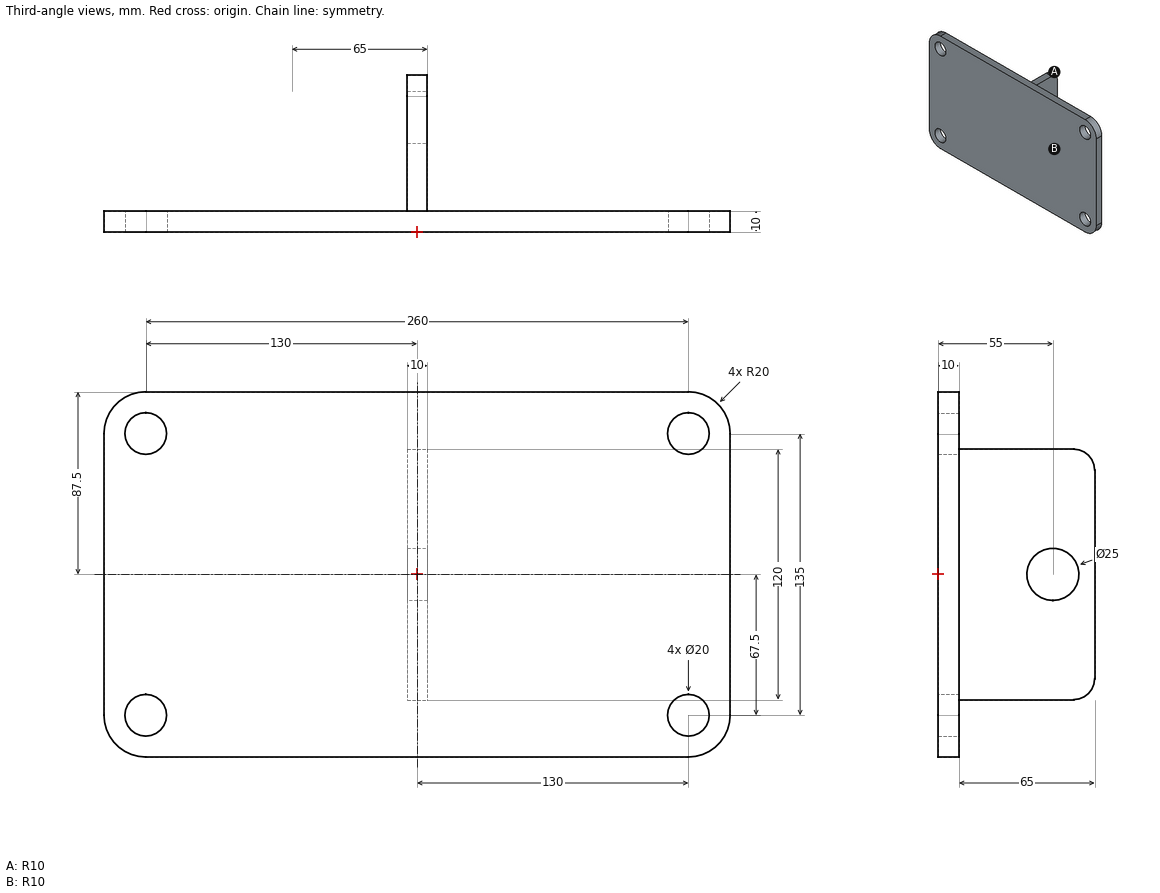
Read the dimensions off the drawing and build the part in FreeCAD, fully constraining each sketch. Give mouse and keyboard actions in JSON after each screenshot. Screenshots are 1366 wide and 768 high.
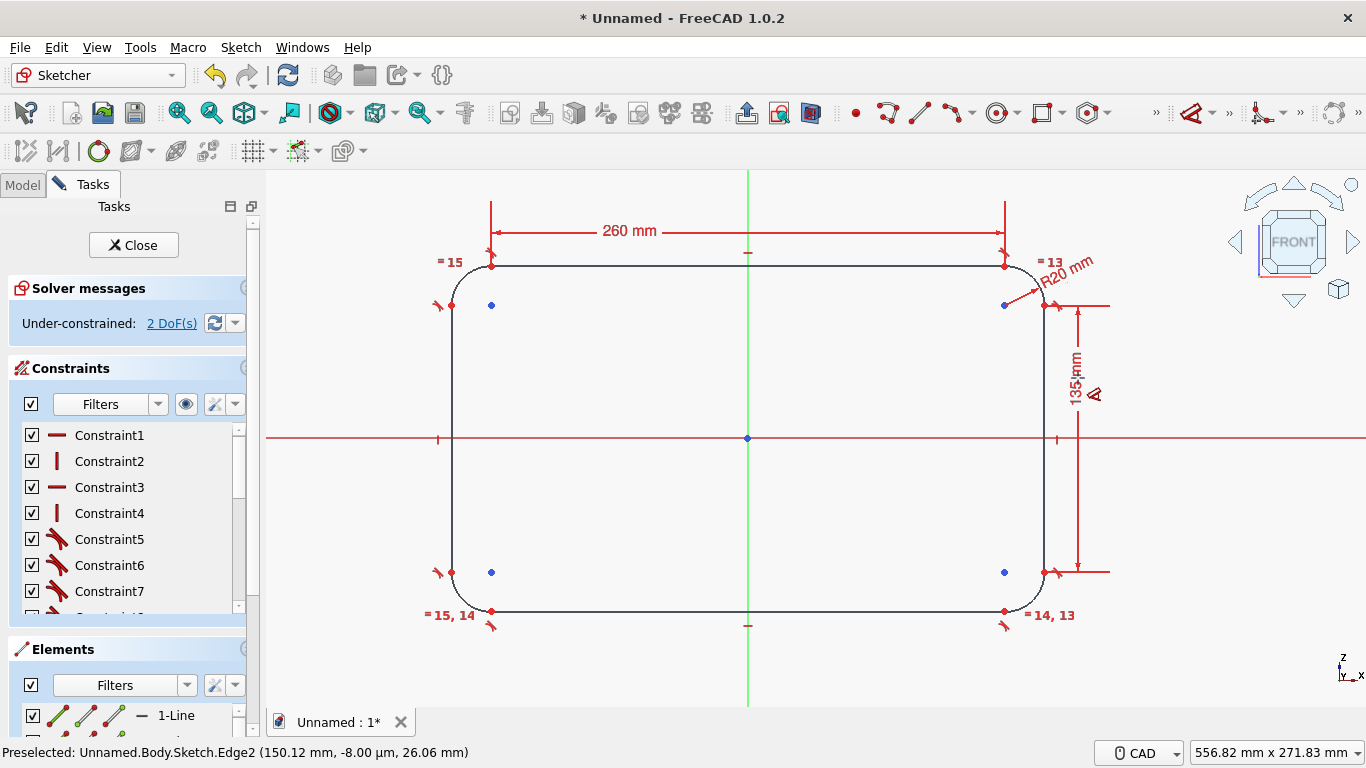
{"action": "left_click", "coordinate": [491, 266]}
{"action": "left_click", "coordinate": [530, 232]}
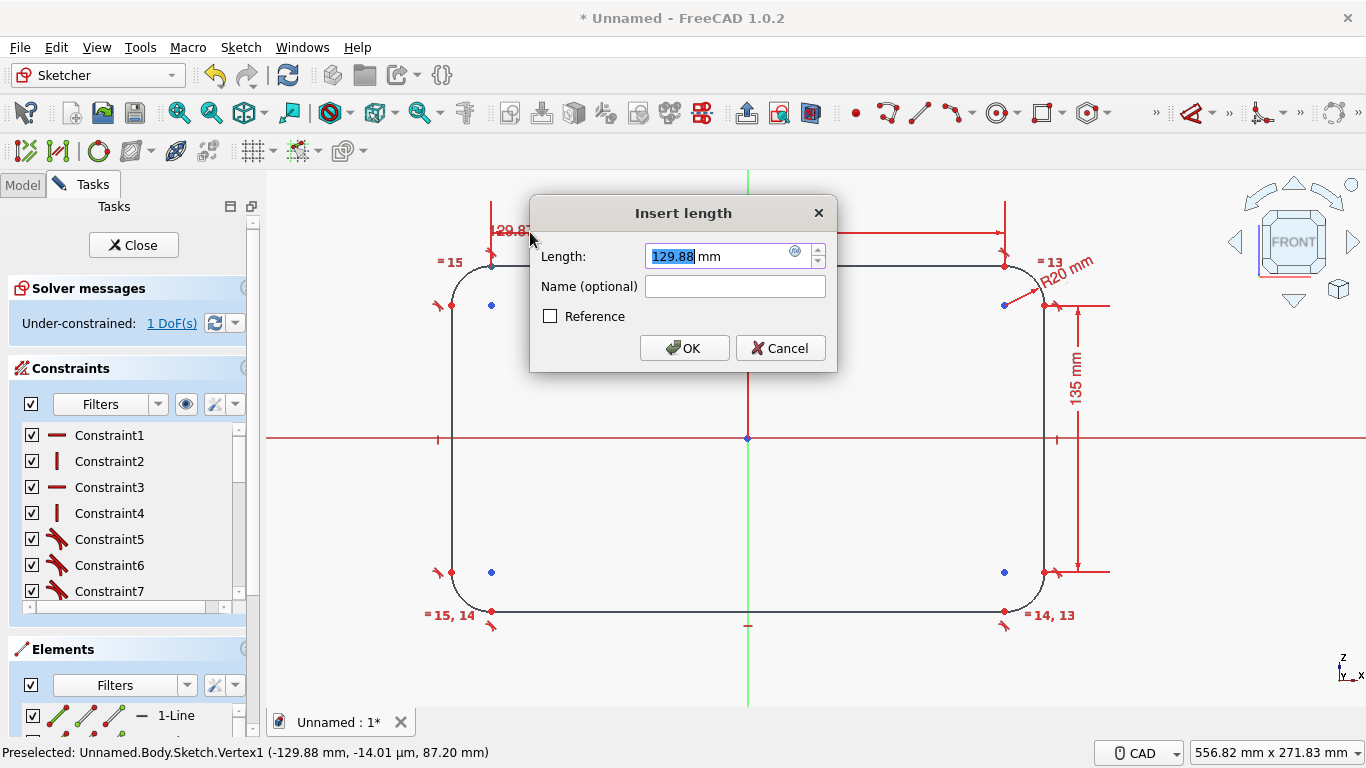
{"action": "type", "text": "130"}
{"action": "key", "text": "Return"}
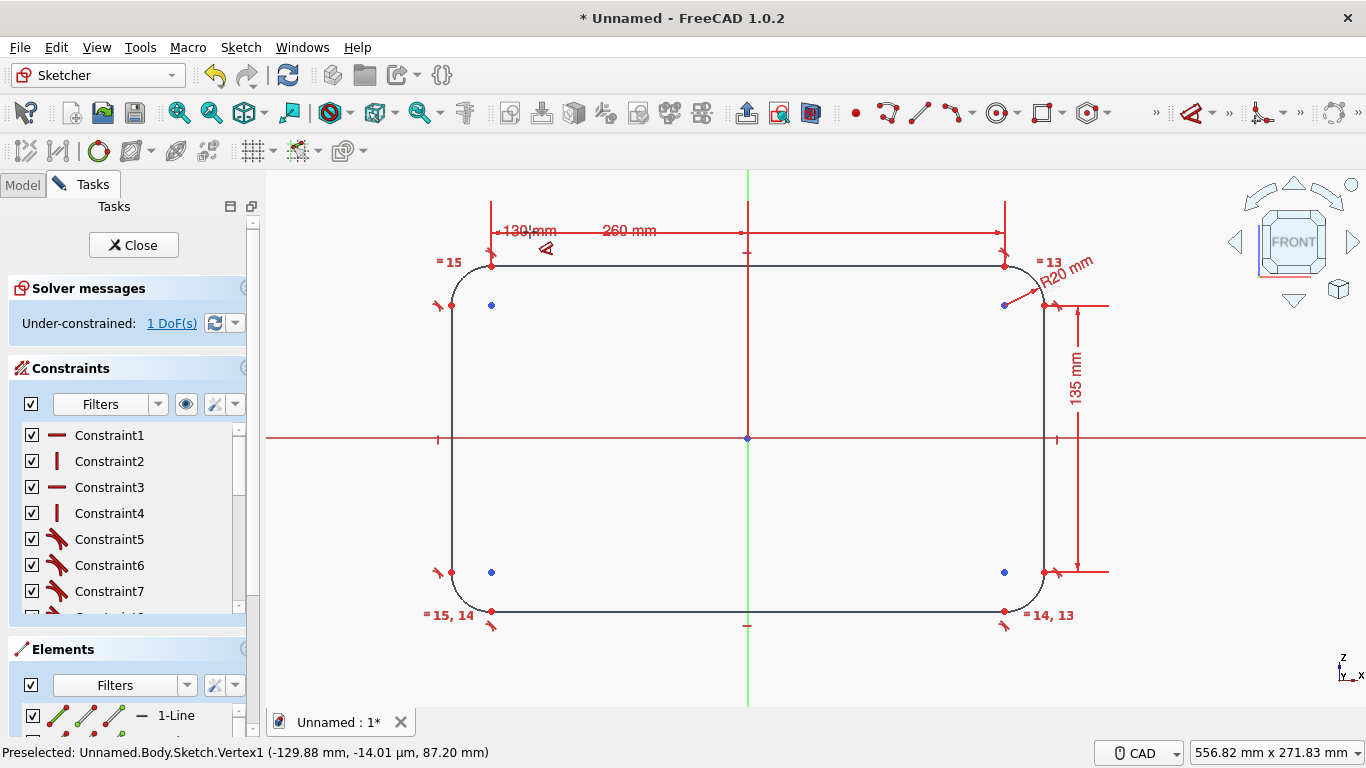
{"action": "left_click", "coordinate": [491, 266]}
{"action": "left_click", "coordinate": [782, 352]}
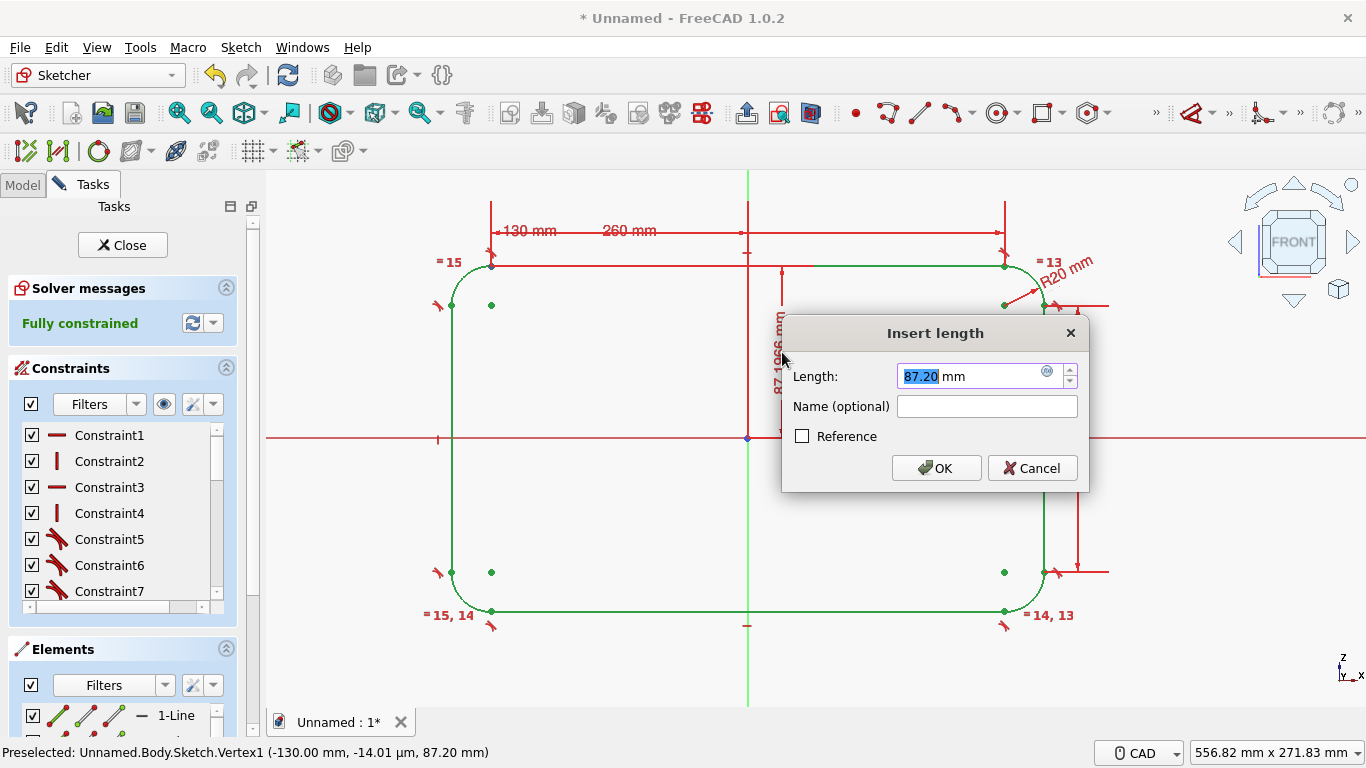
{"action": "type", "text": "87.5"}
{"action": "key", "text": "Return"}
{"action": "key", "text": "Escape"}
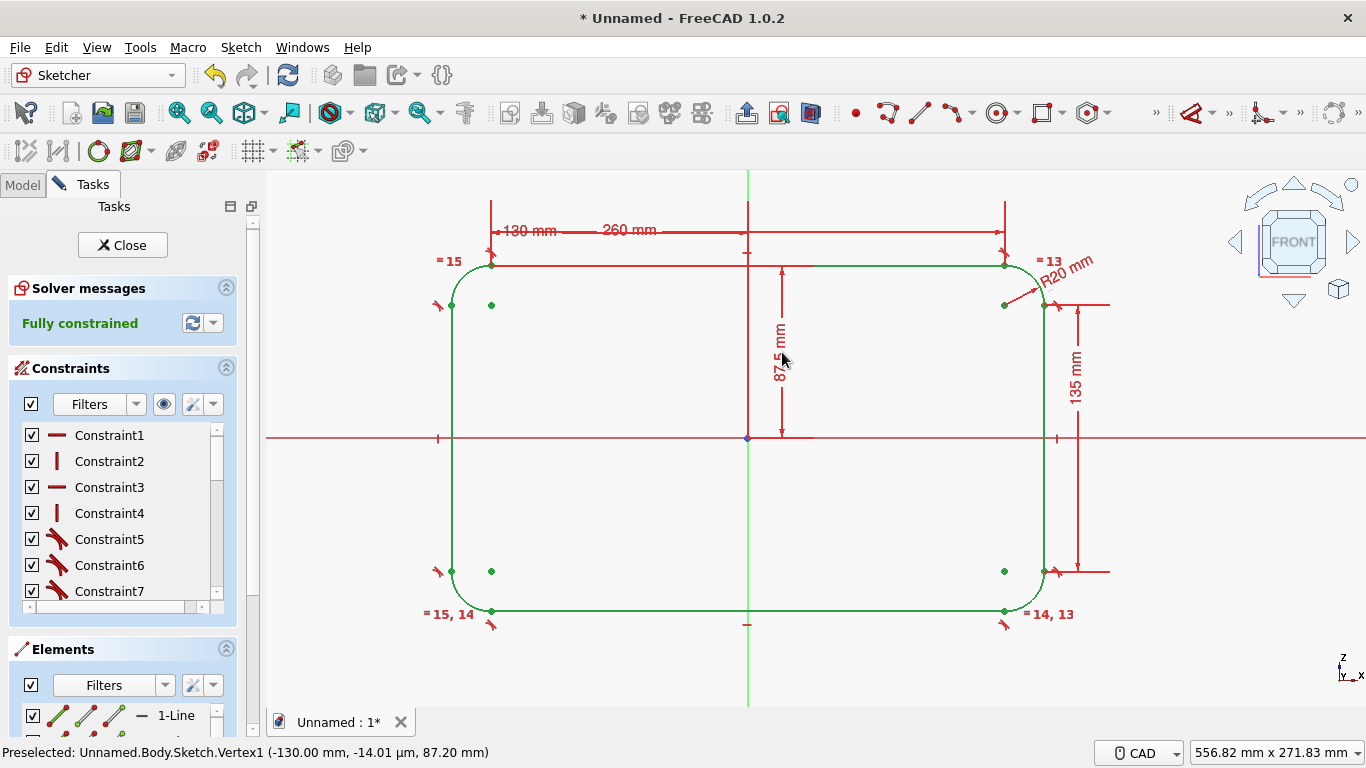
{"action": "left_click", "coordinate": [123, 245]}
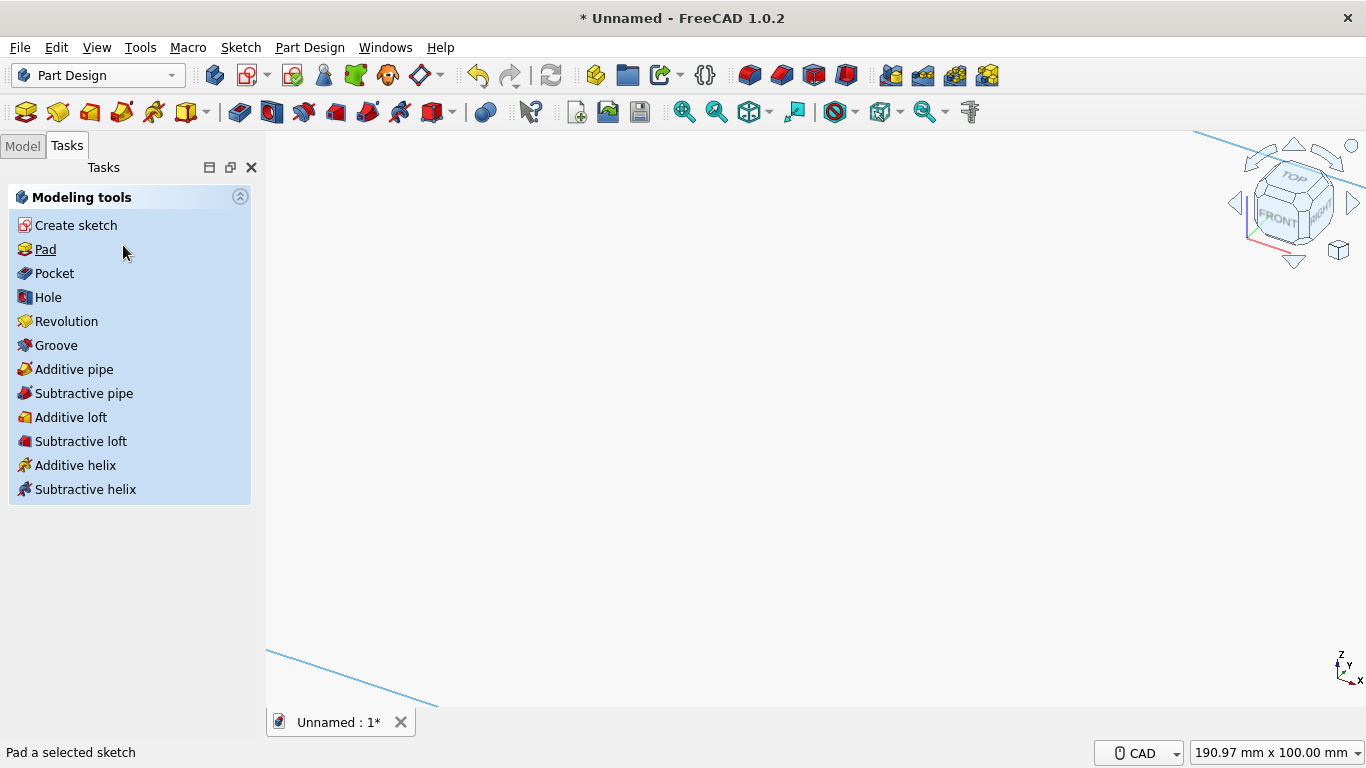
{"action": "left_click", "coordinate": [26, 112]}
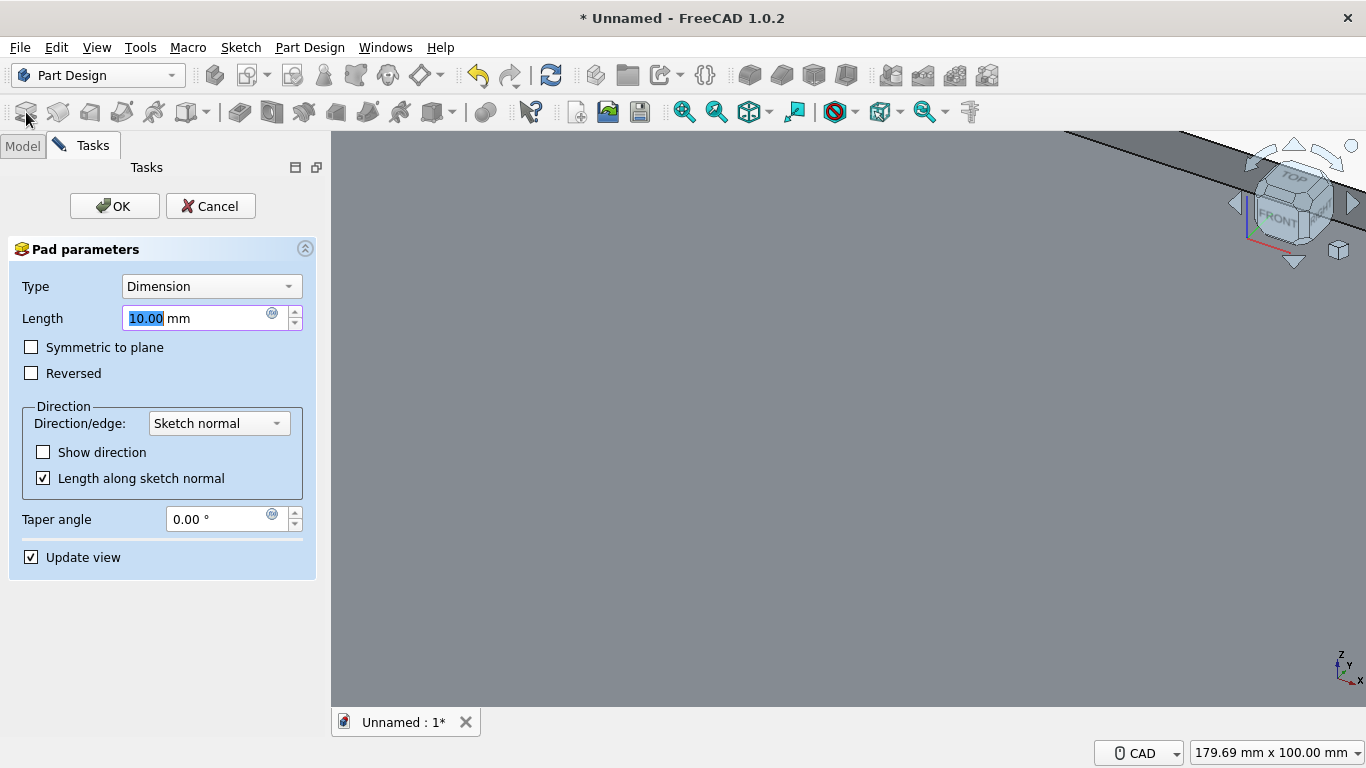
{"action": "type", "text": "10"}
{"action": "key", "text": "Tab"}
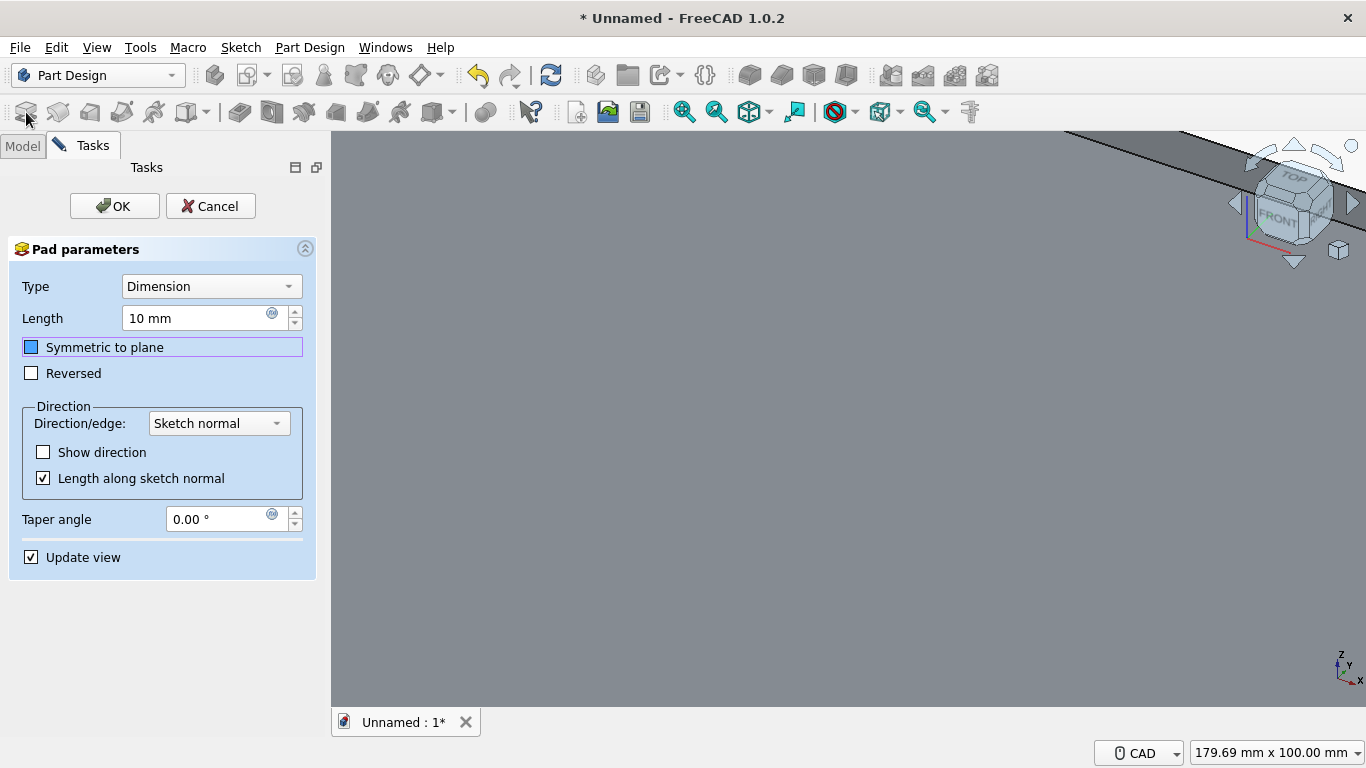
{"action": "left_click", "coordinate": [30, 373]}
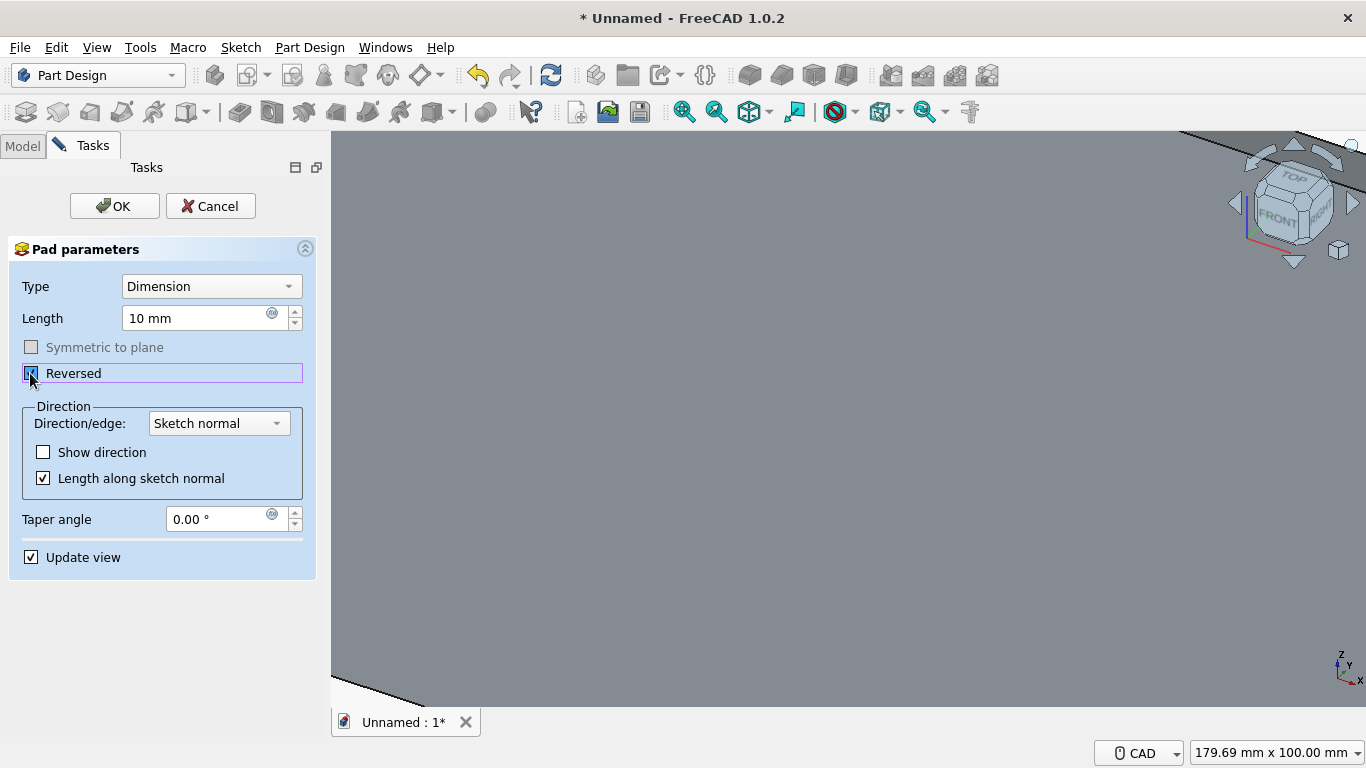
{"action": "left_click", "coordinate": [115, 206]}